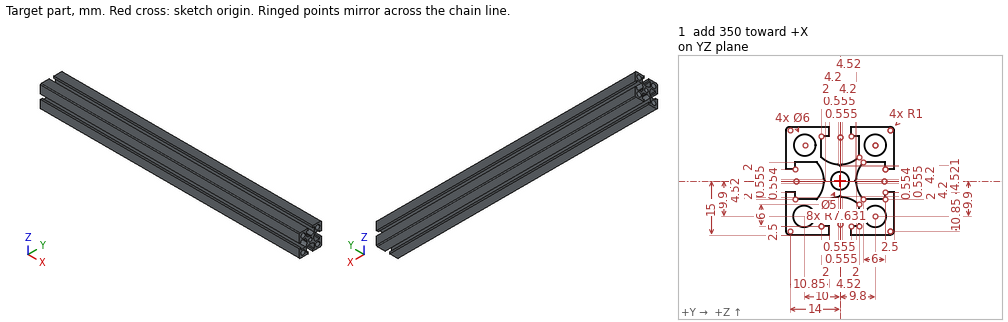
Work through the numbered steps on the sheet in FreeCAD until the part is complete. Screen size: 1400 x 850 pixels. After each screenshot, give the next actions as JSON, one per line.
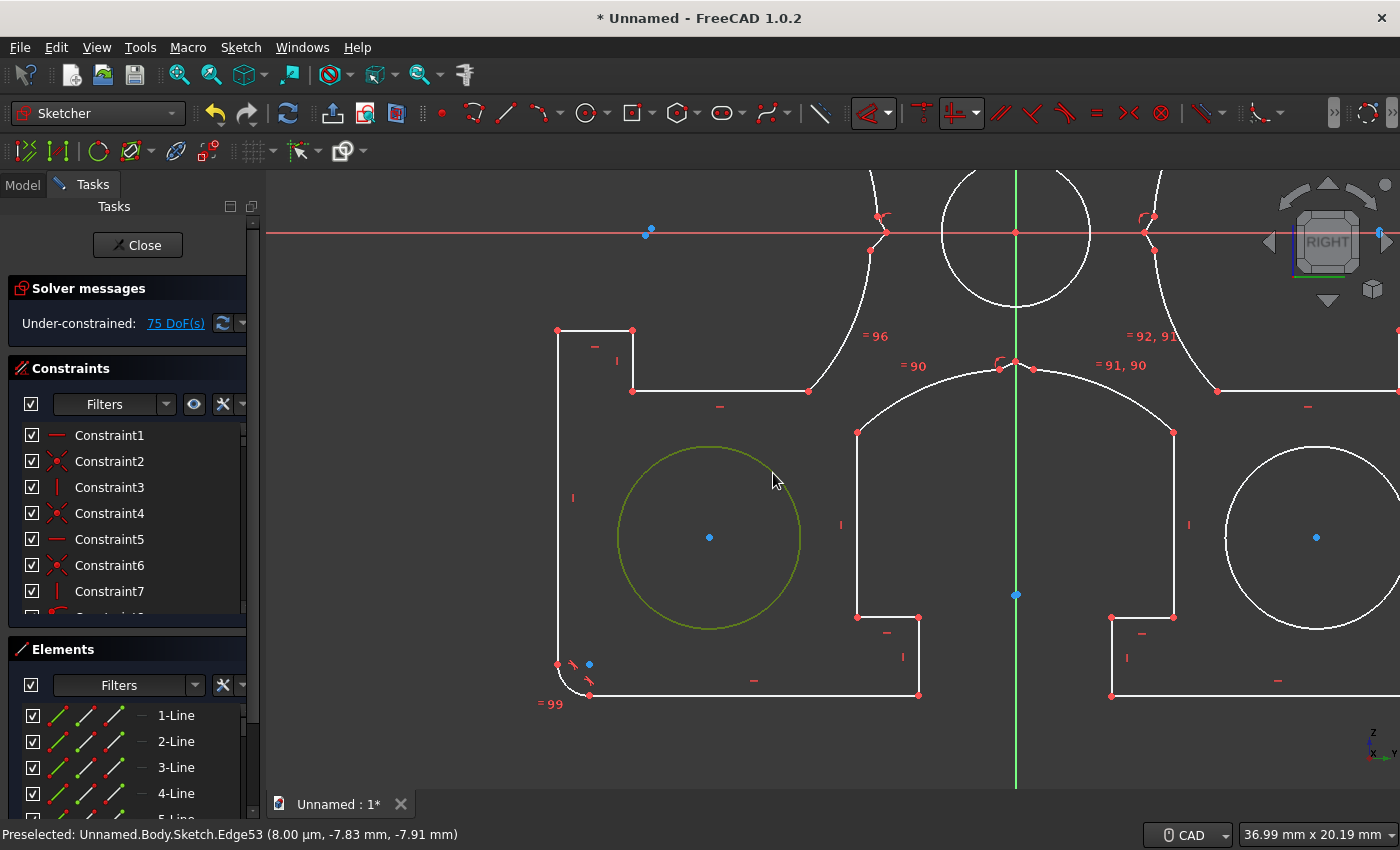
{"action": "left_click", "coordinate": [1225, 535]}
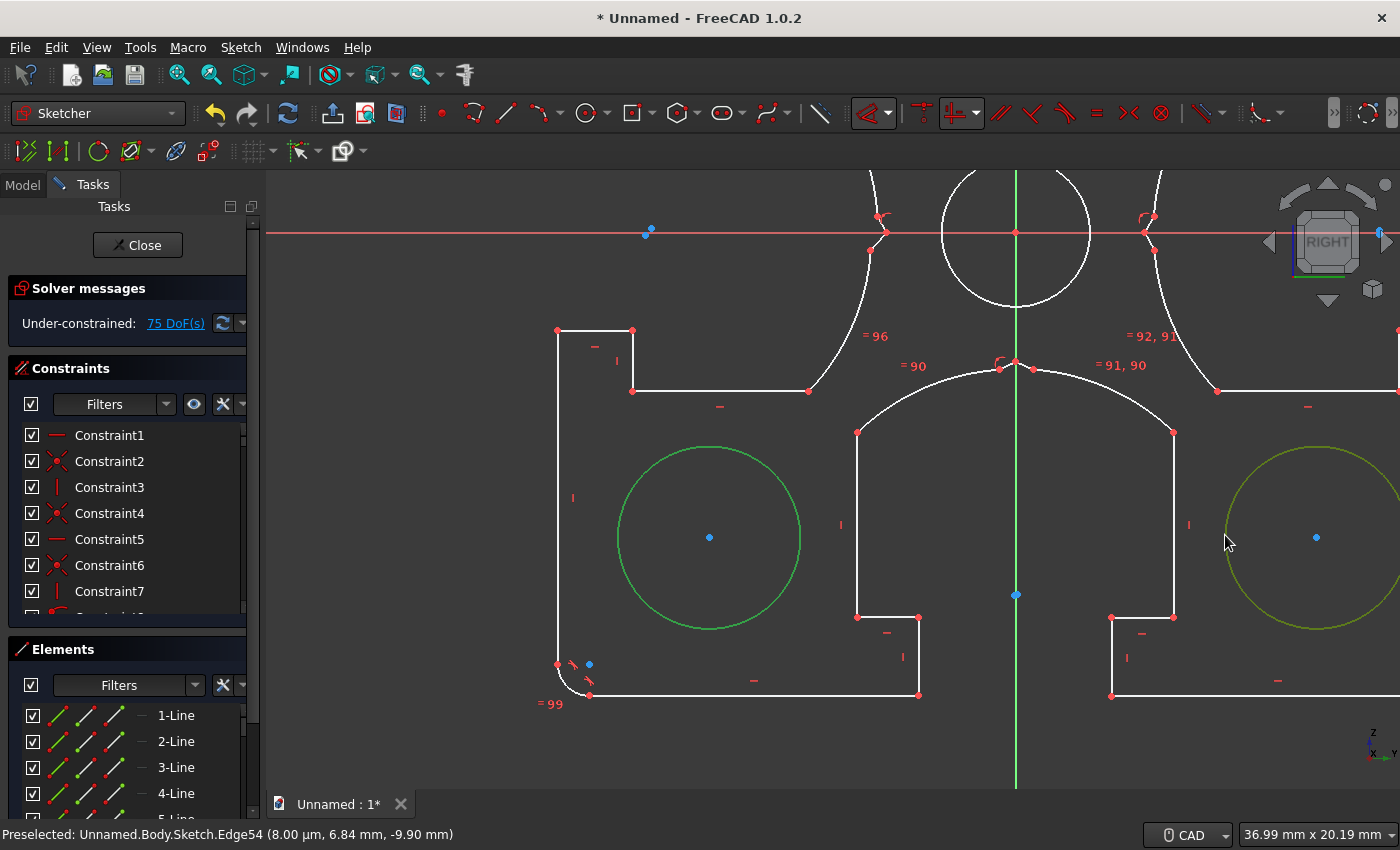
{"action": "scroll", "coordinate": [559, 681], "scroll_direction": "down", "scroll_amount": 4}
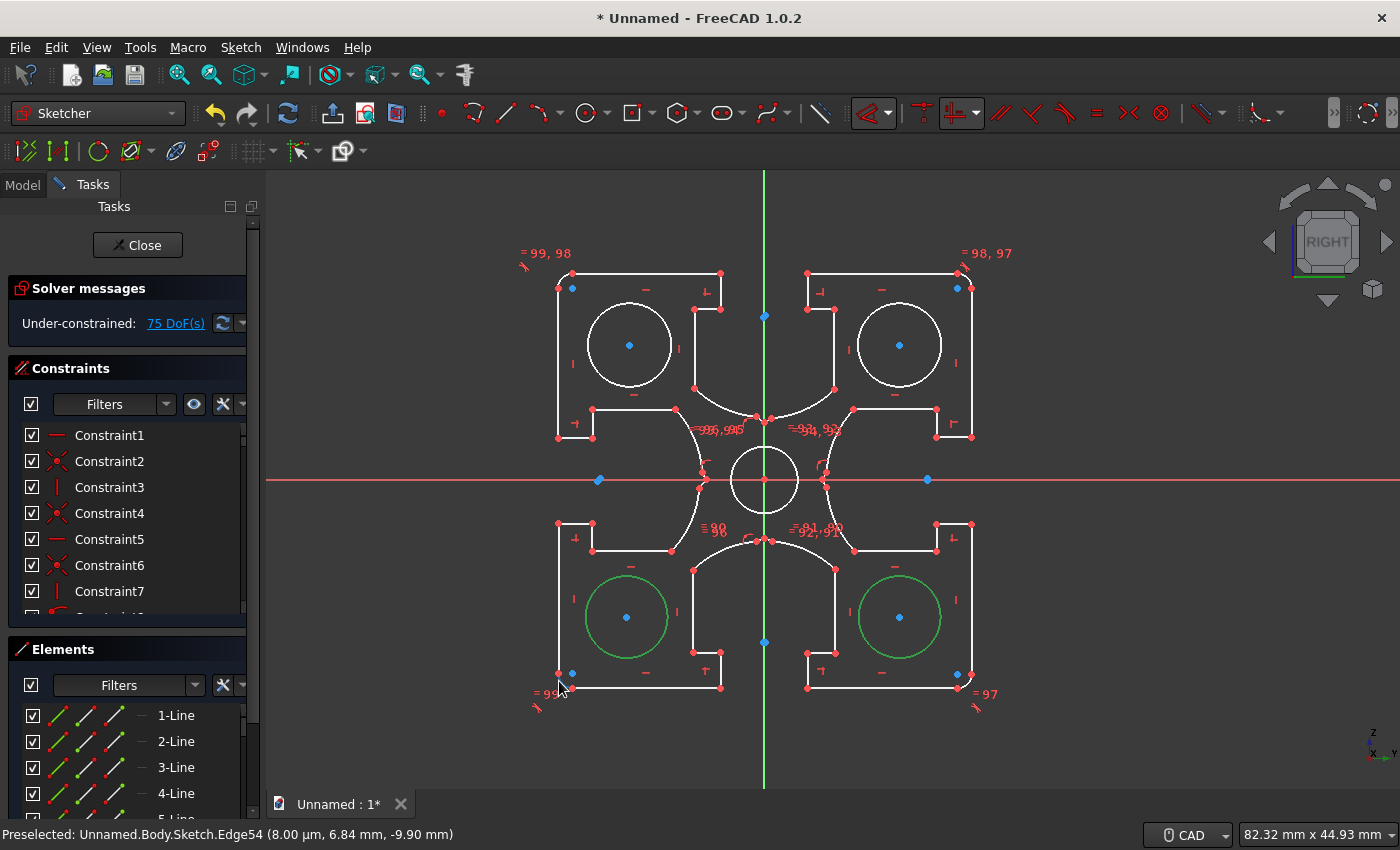
{"action": "left_click", "coordinate": [659, 315]}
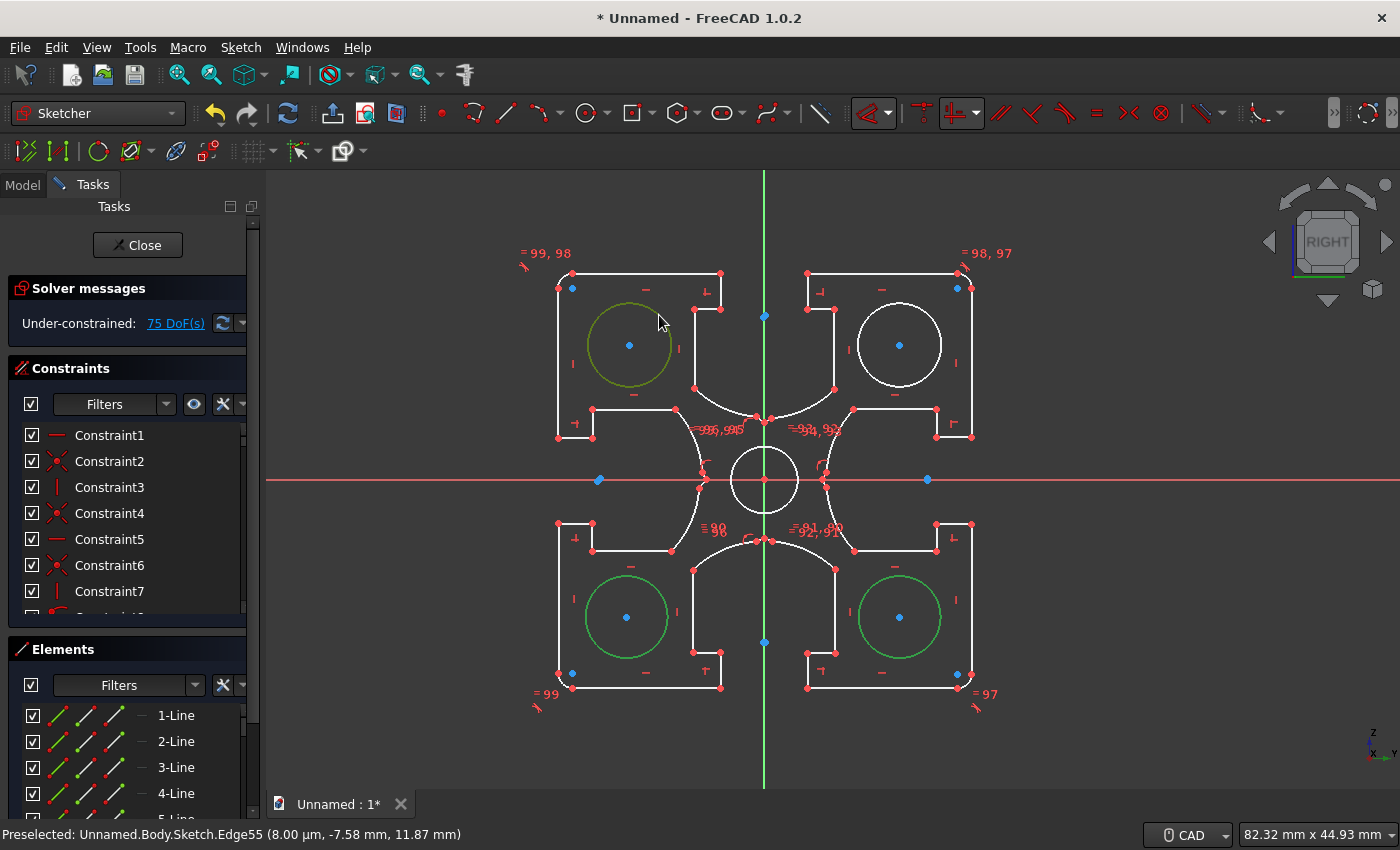
{"action": "left_click", "coordinate": [929, 315]}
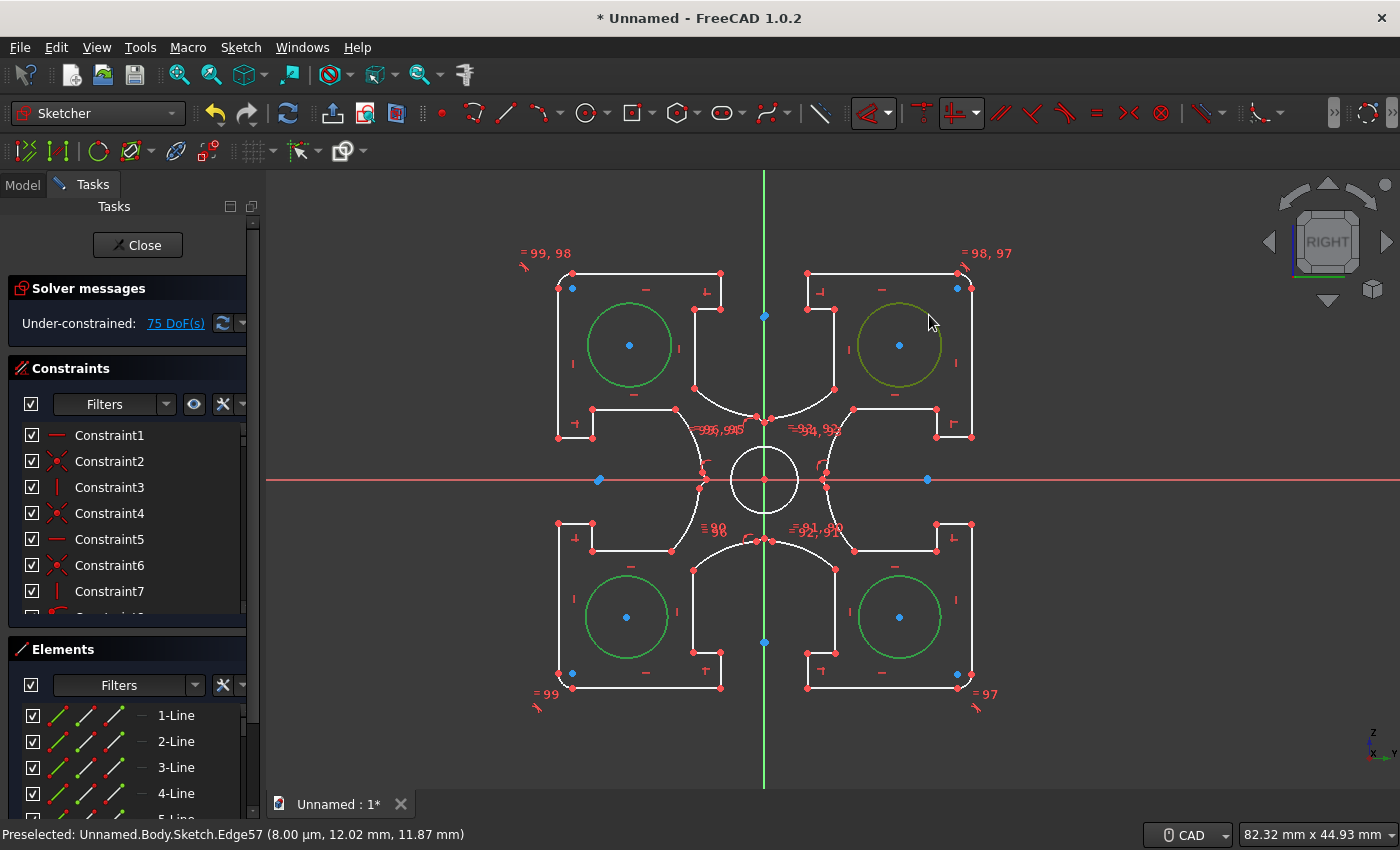
{"action": "key", "text": "e"}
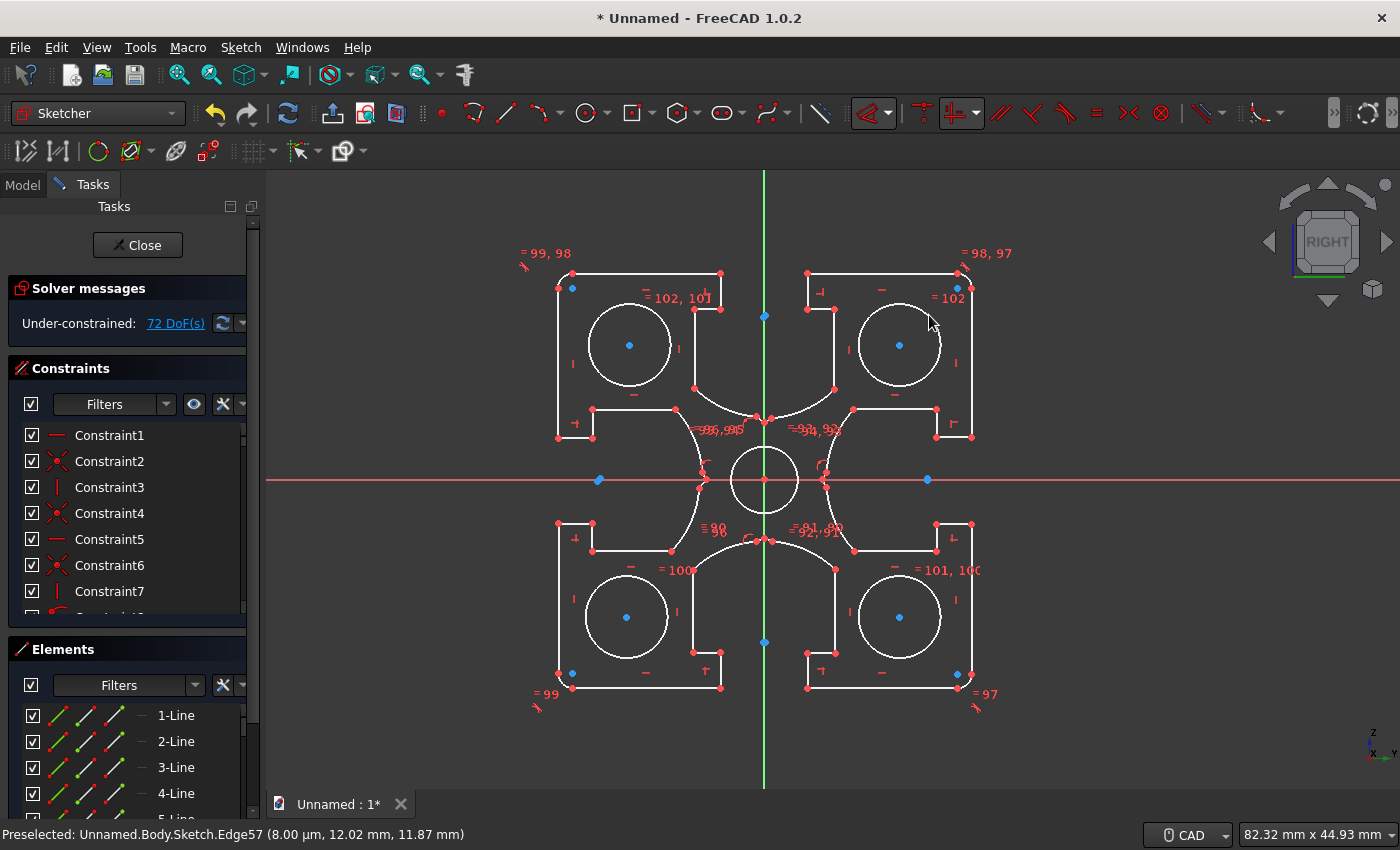
{"action": "scroll", "coordinate": [764, 643], "scroll_direction": "up", "scroll_amount": 11}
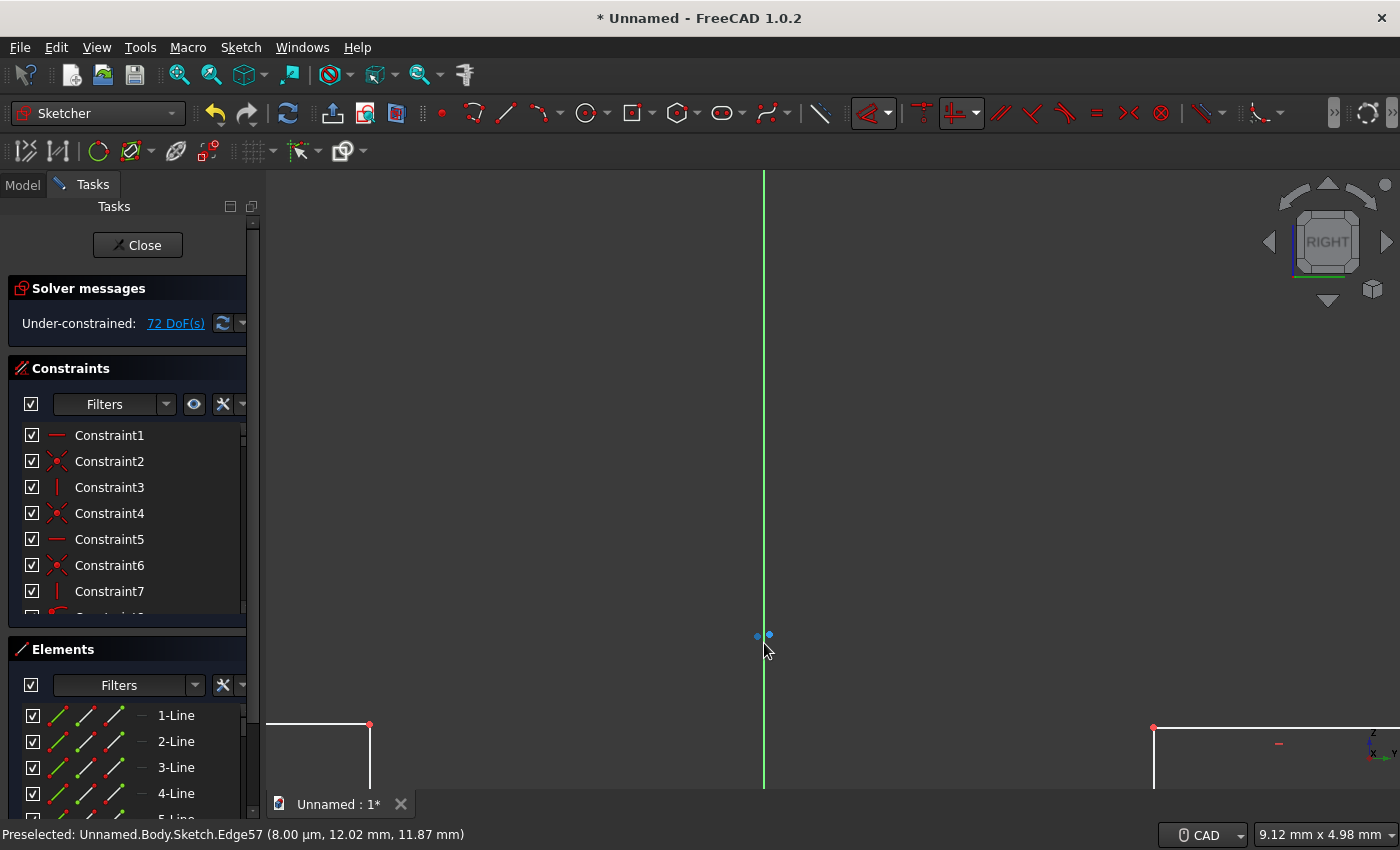
{"action": "left_click", "coordinate": [758, 636]}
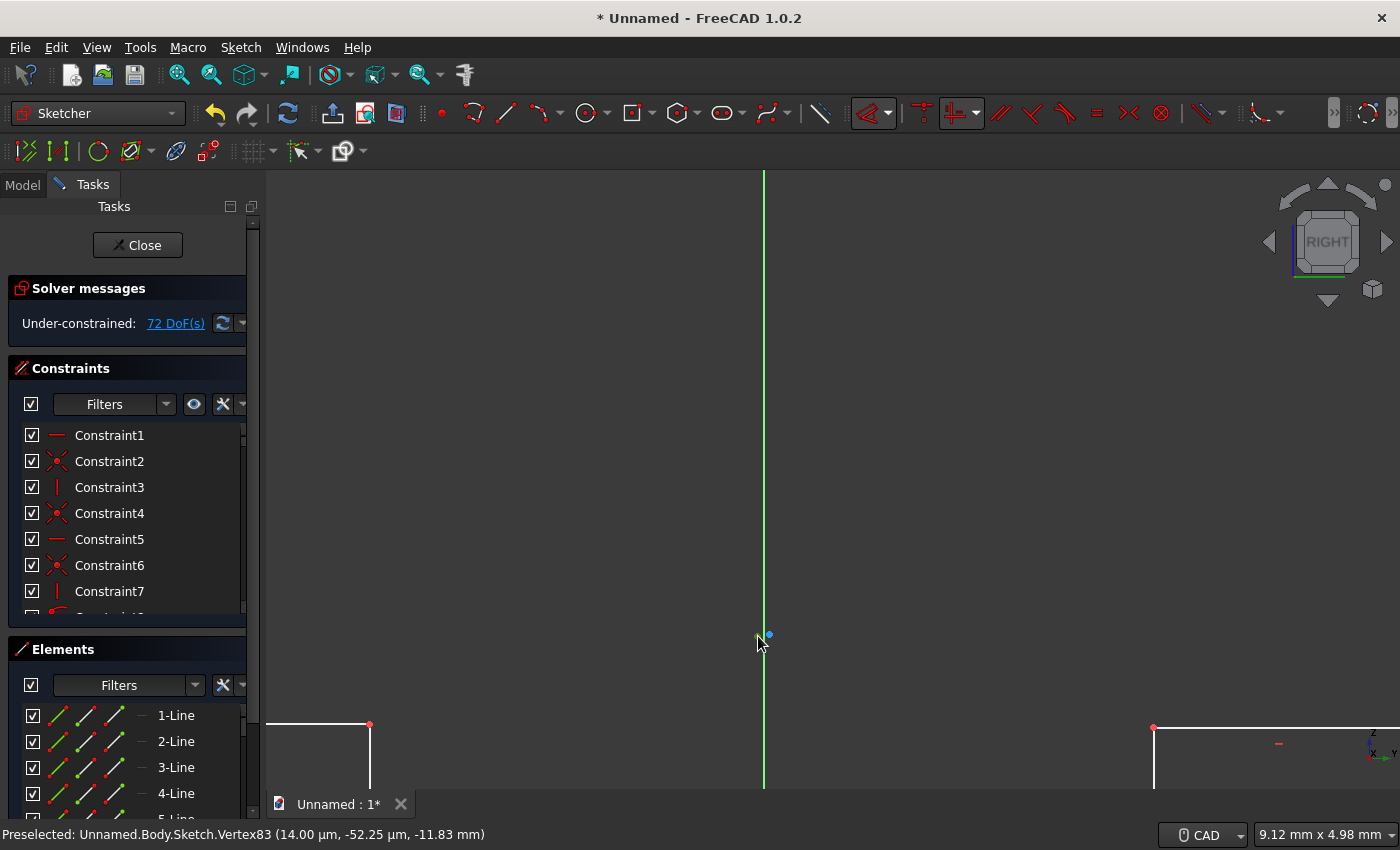
{"action": "left_click", "coordinate": [770, 635]}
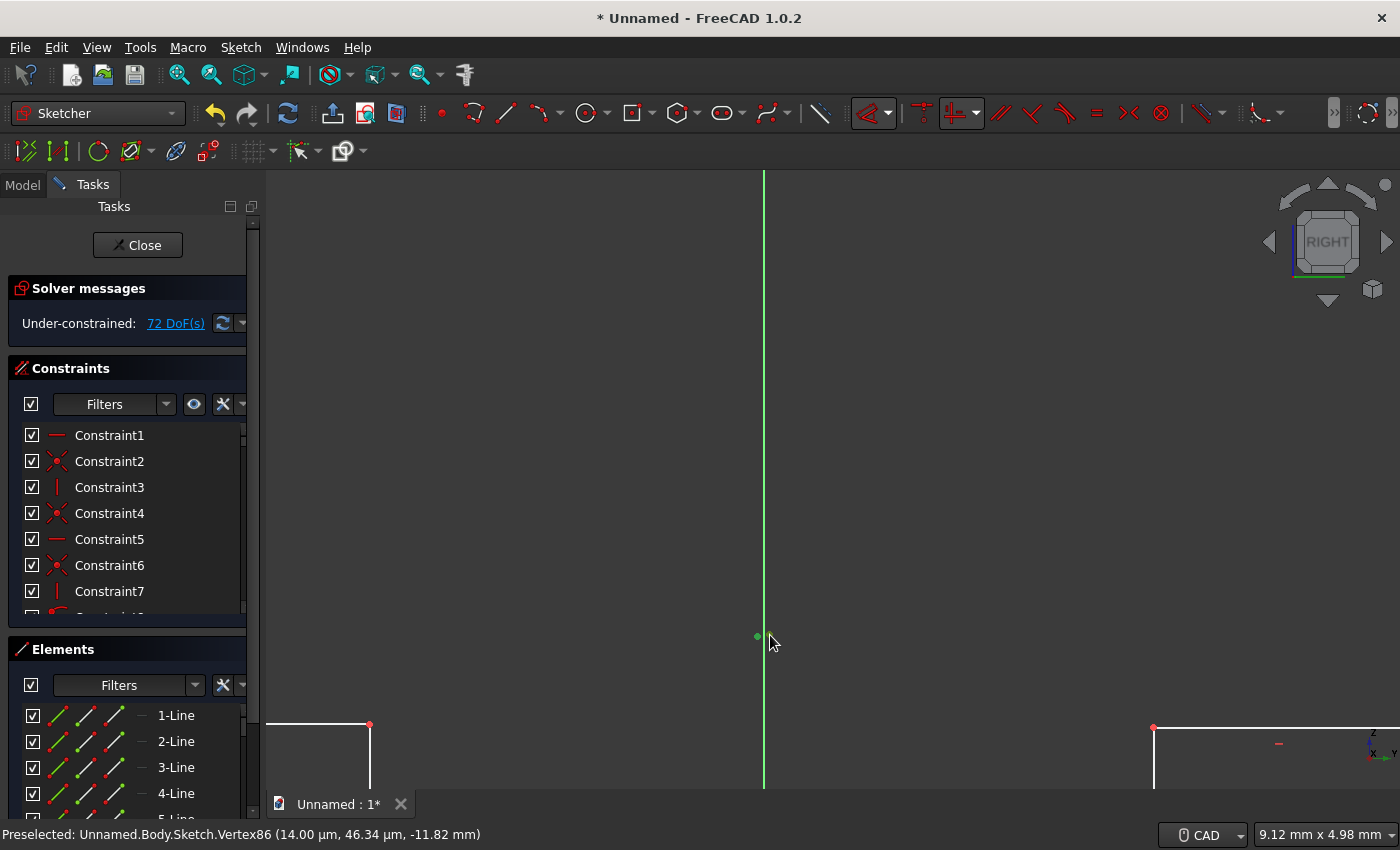
{"action": "left_click", "coordinate": [764, 721]}